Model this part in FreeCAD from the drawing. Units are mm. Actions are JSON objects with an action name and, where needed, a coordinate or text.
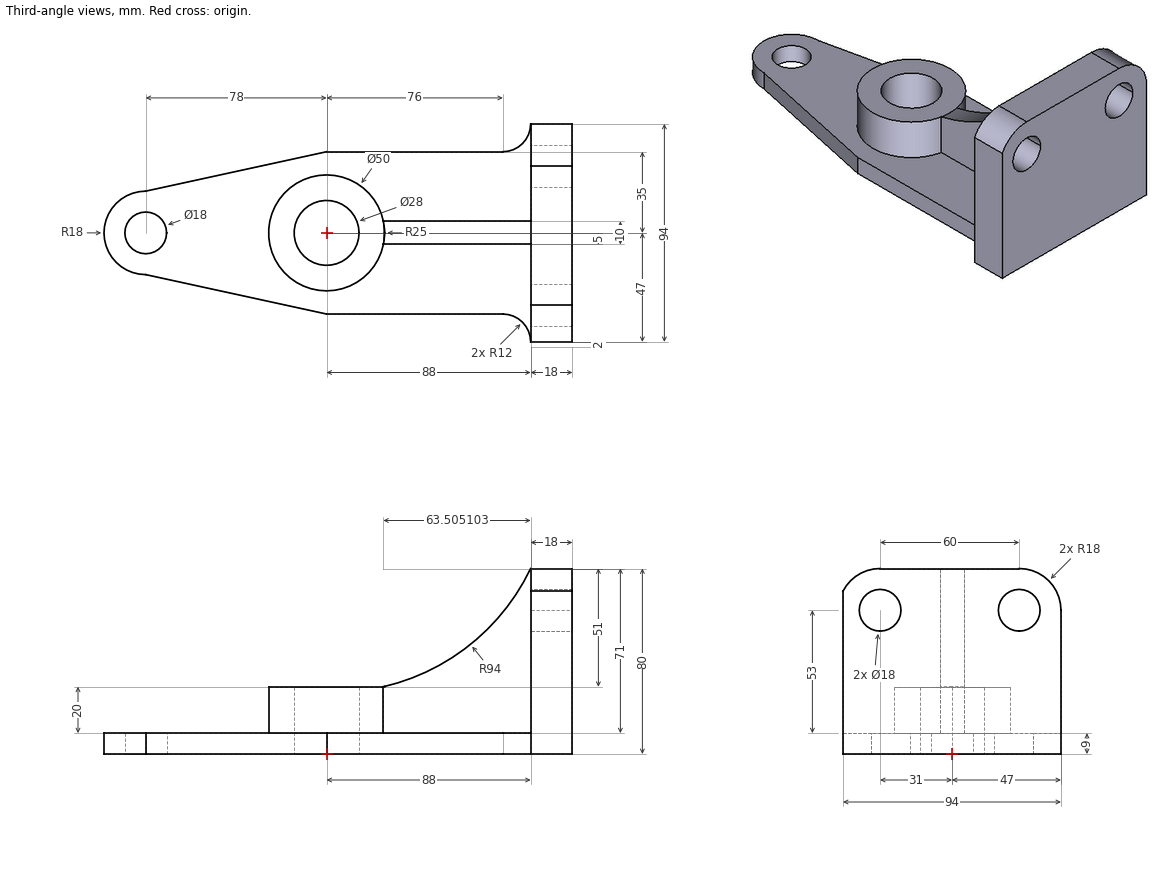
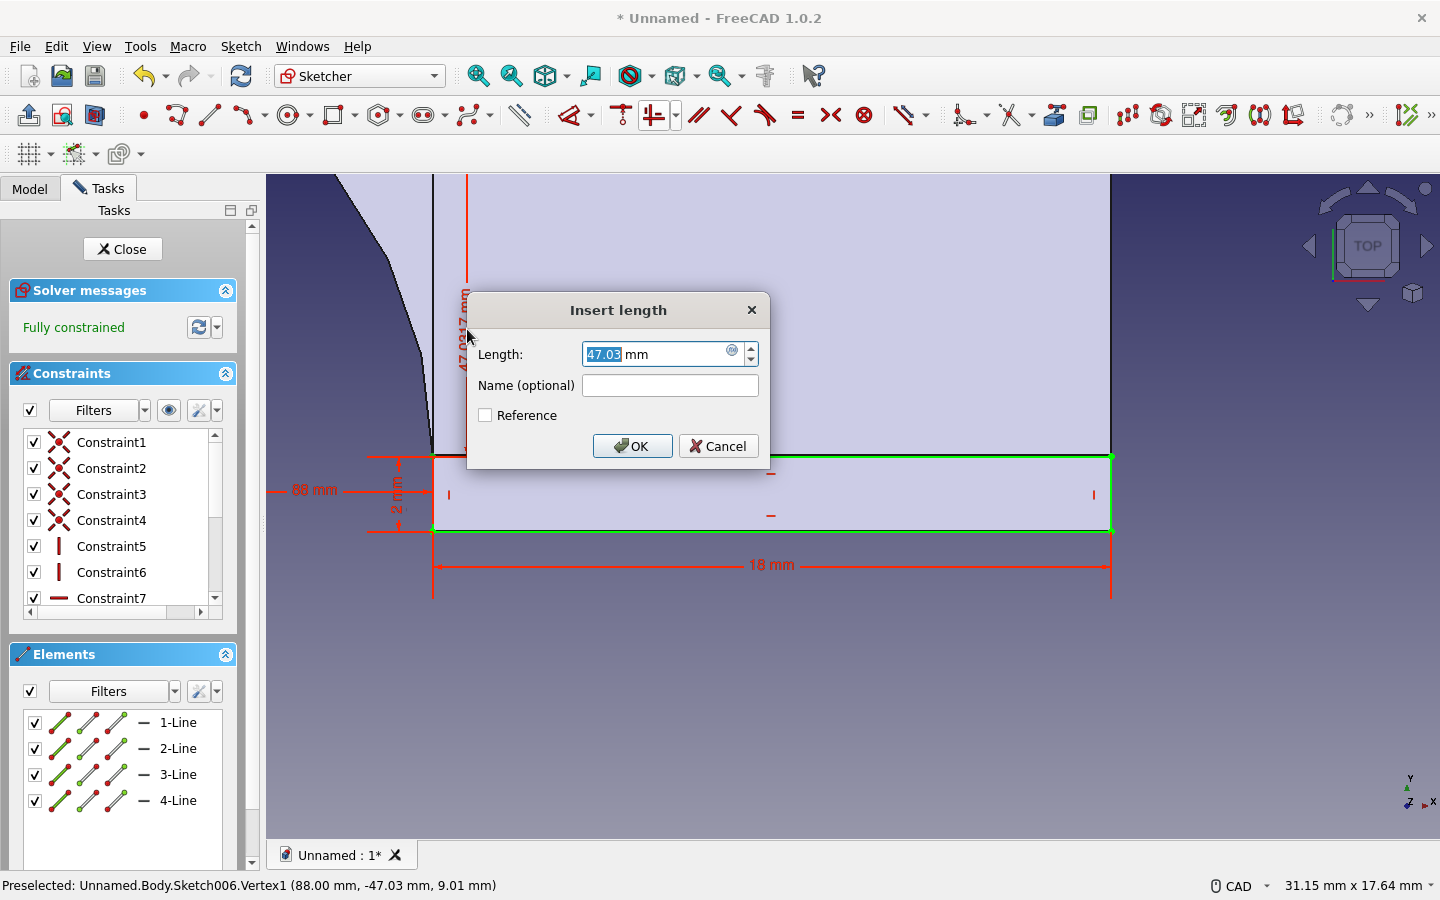
{"action": "type", "text": "47"}
{"action": "key", "text": "Return"}
{"action": "key", "text": "Escape"}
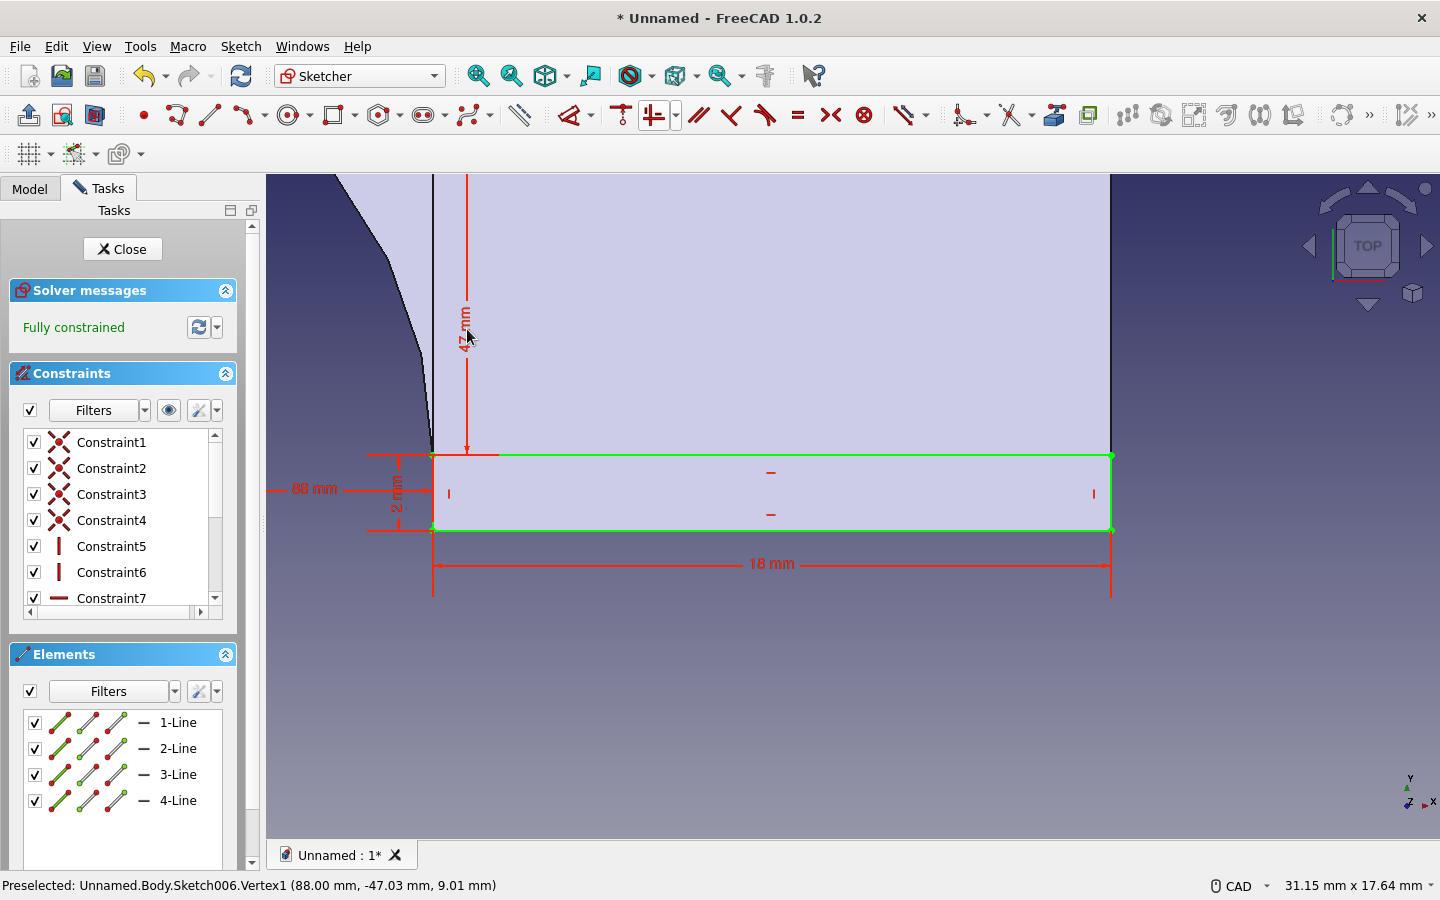
{"action": "left_click", "coordinate": [123, 249]}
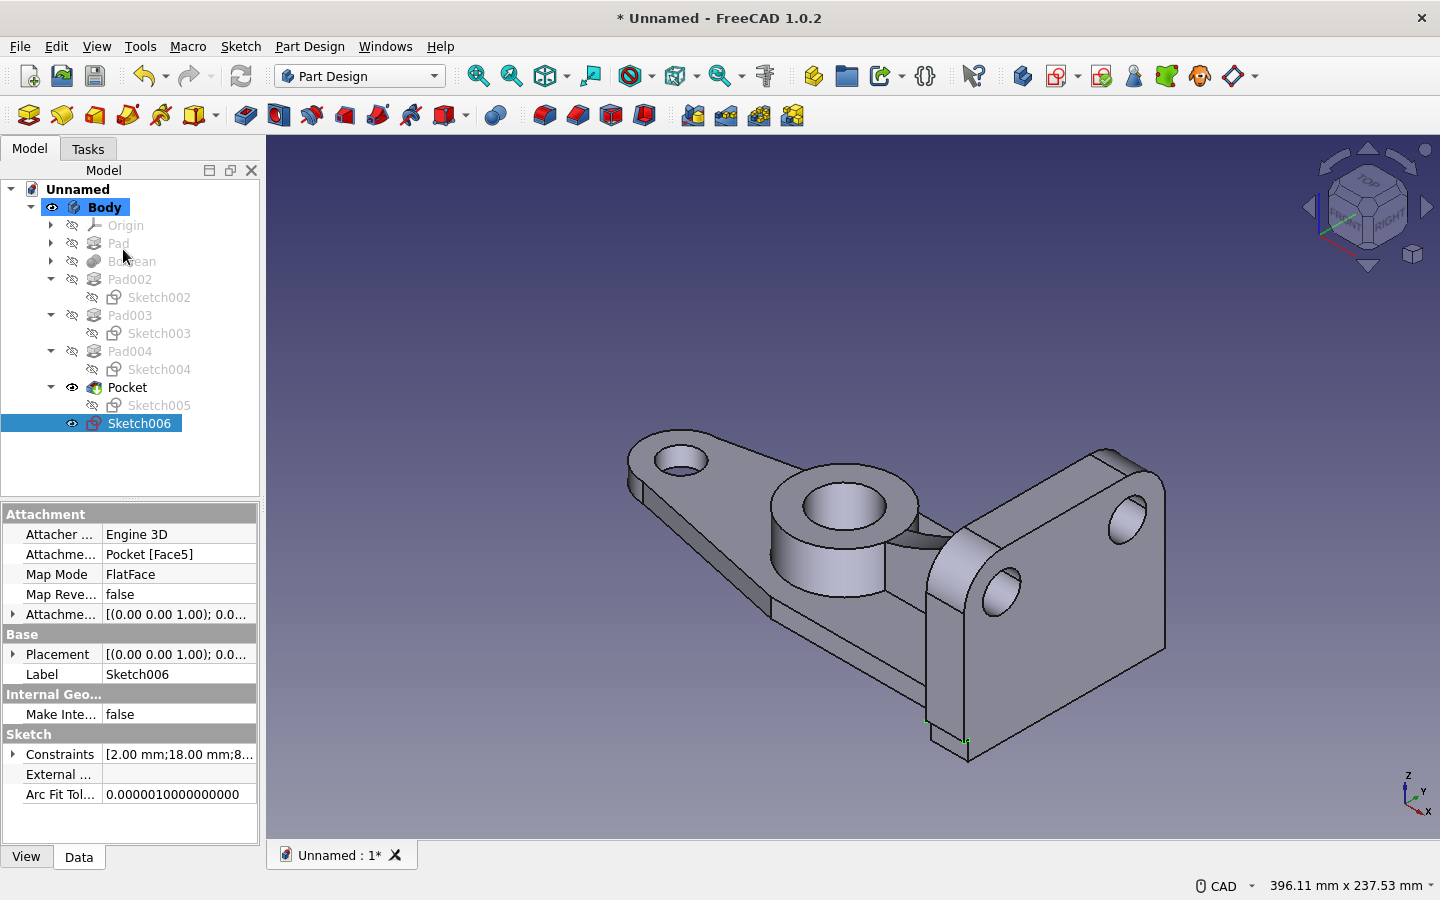
{"action": "left_click", "coordinate": [246, 116]}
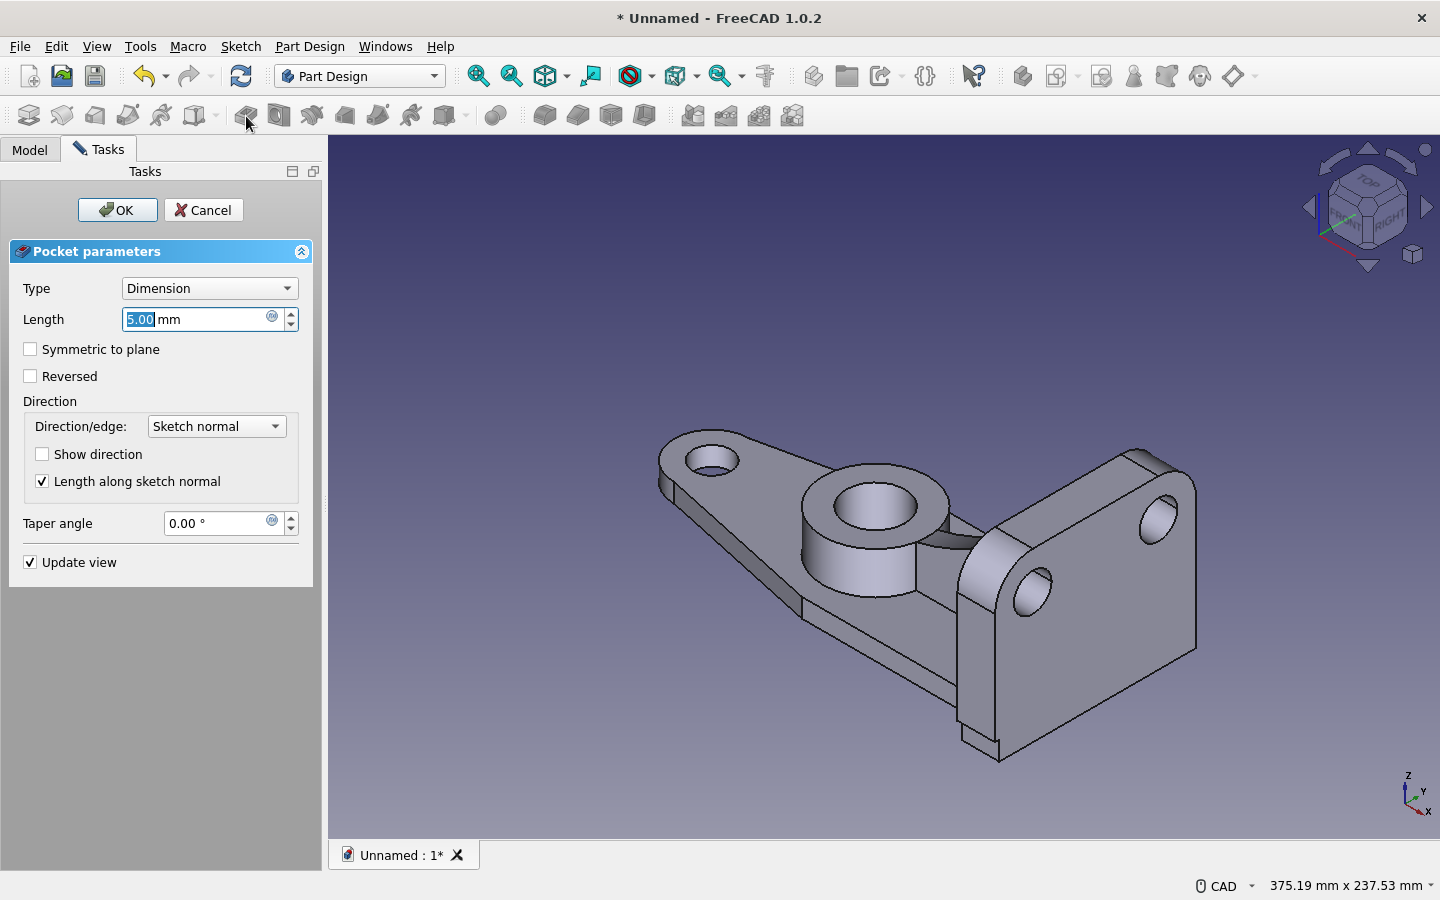
{"action": "left_click", "coordinate": [210, 288]}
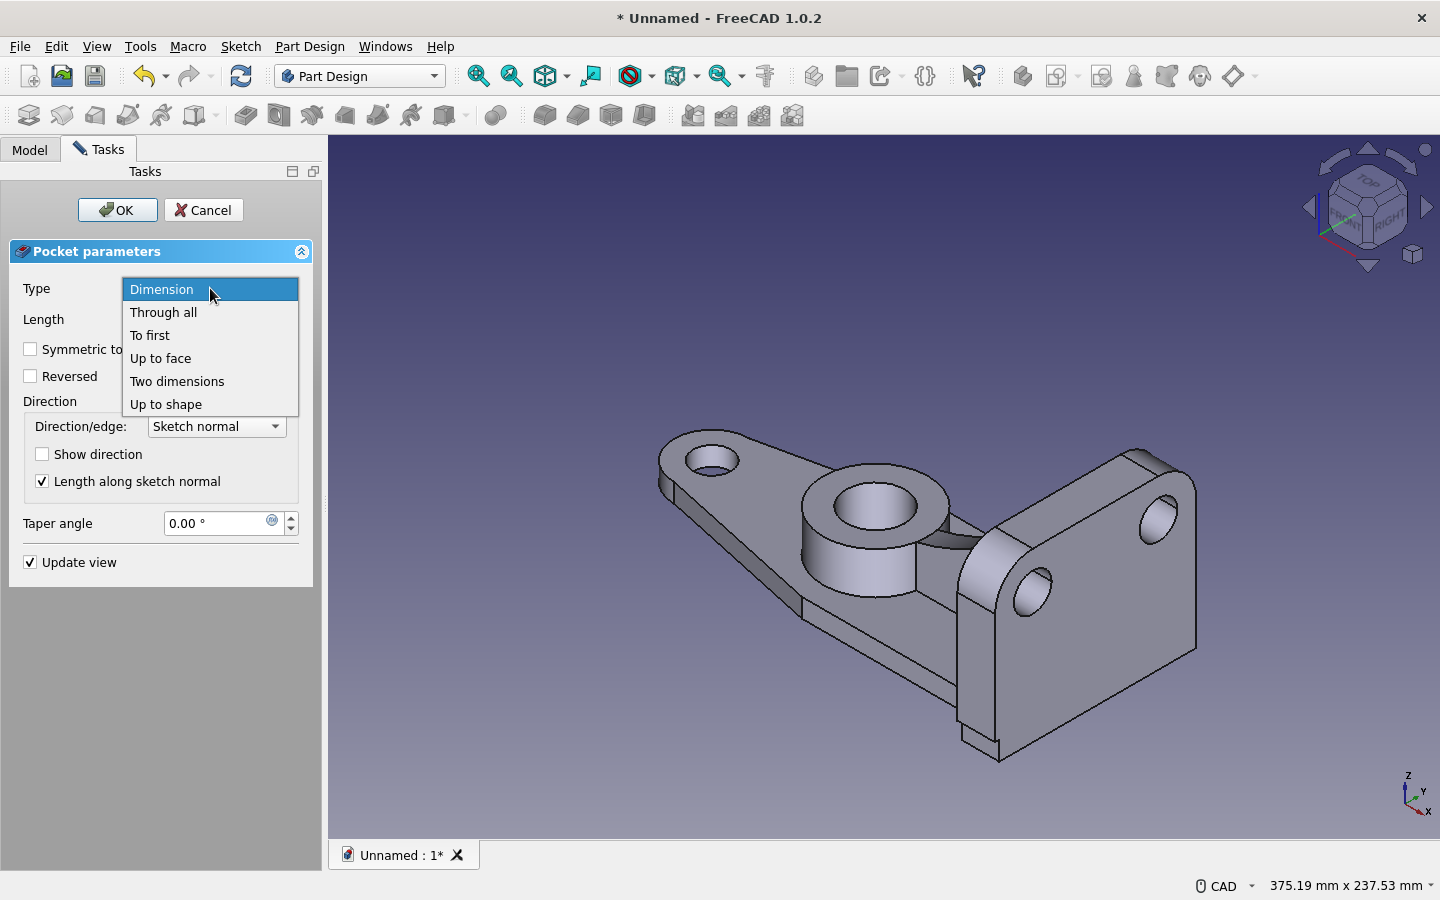
{"action": "left_click", "coordinate": [208, 312]}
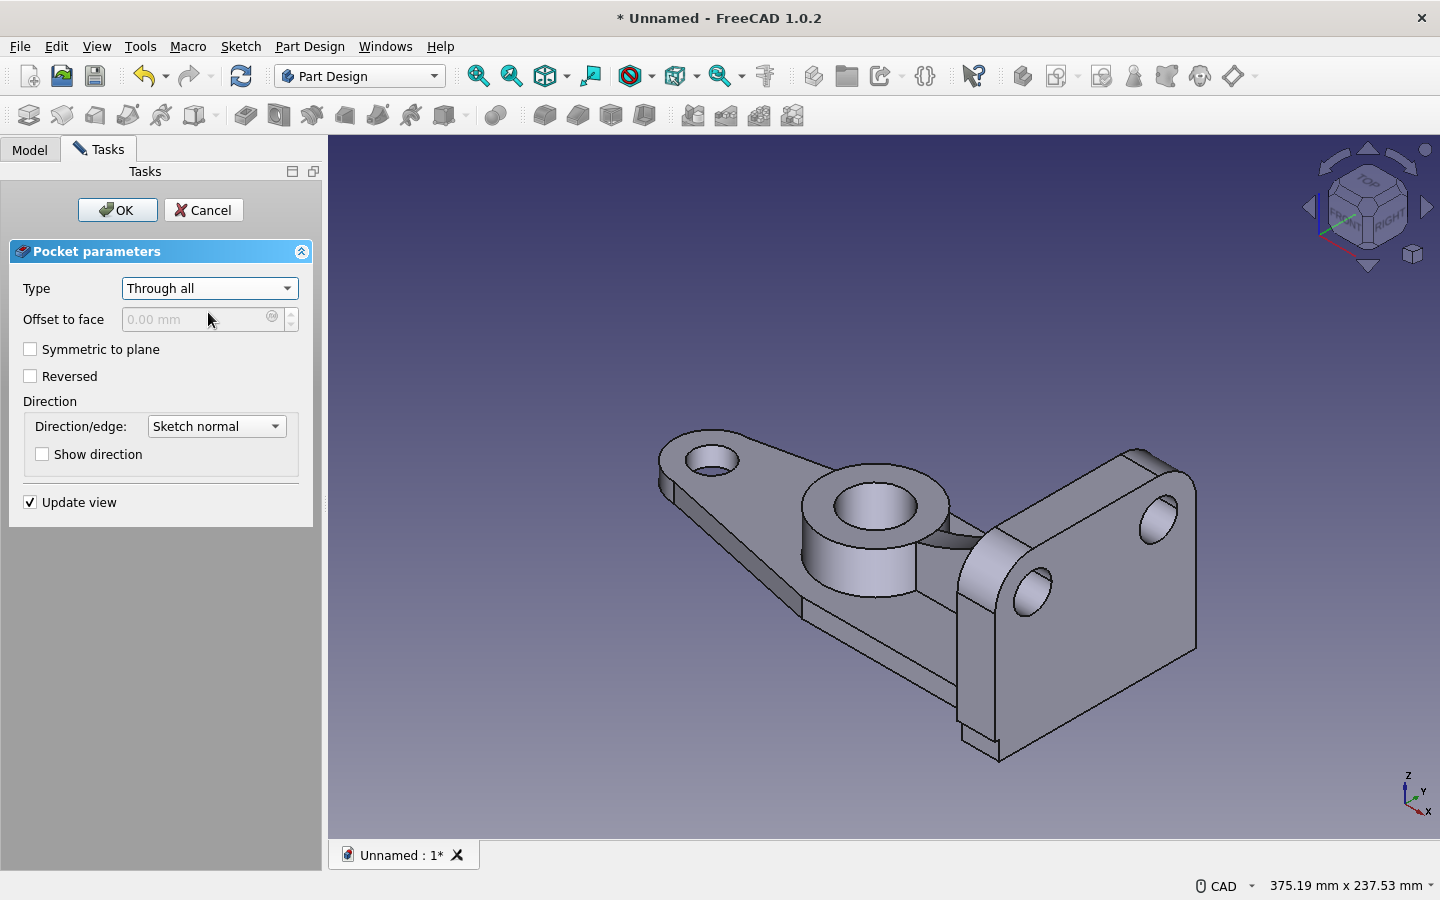
{"action": "left_click", "coordinate": [31, 376]}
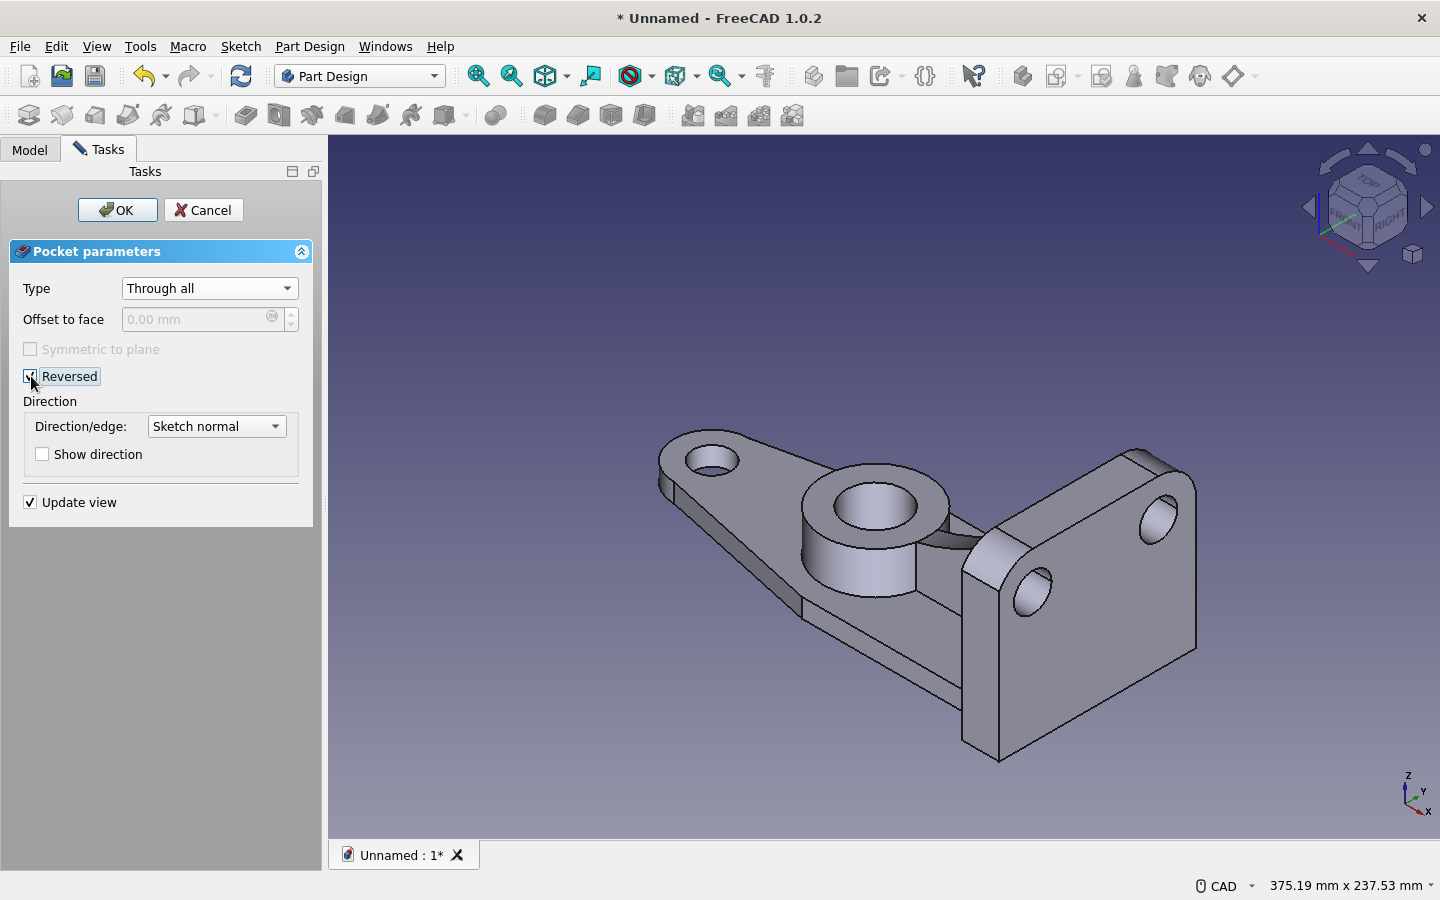
{"action": "left_click", "coordinate": [118, 210]}